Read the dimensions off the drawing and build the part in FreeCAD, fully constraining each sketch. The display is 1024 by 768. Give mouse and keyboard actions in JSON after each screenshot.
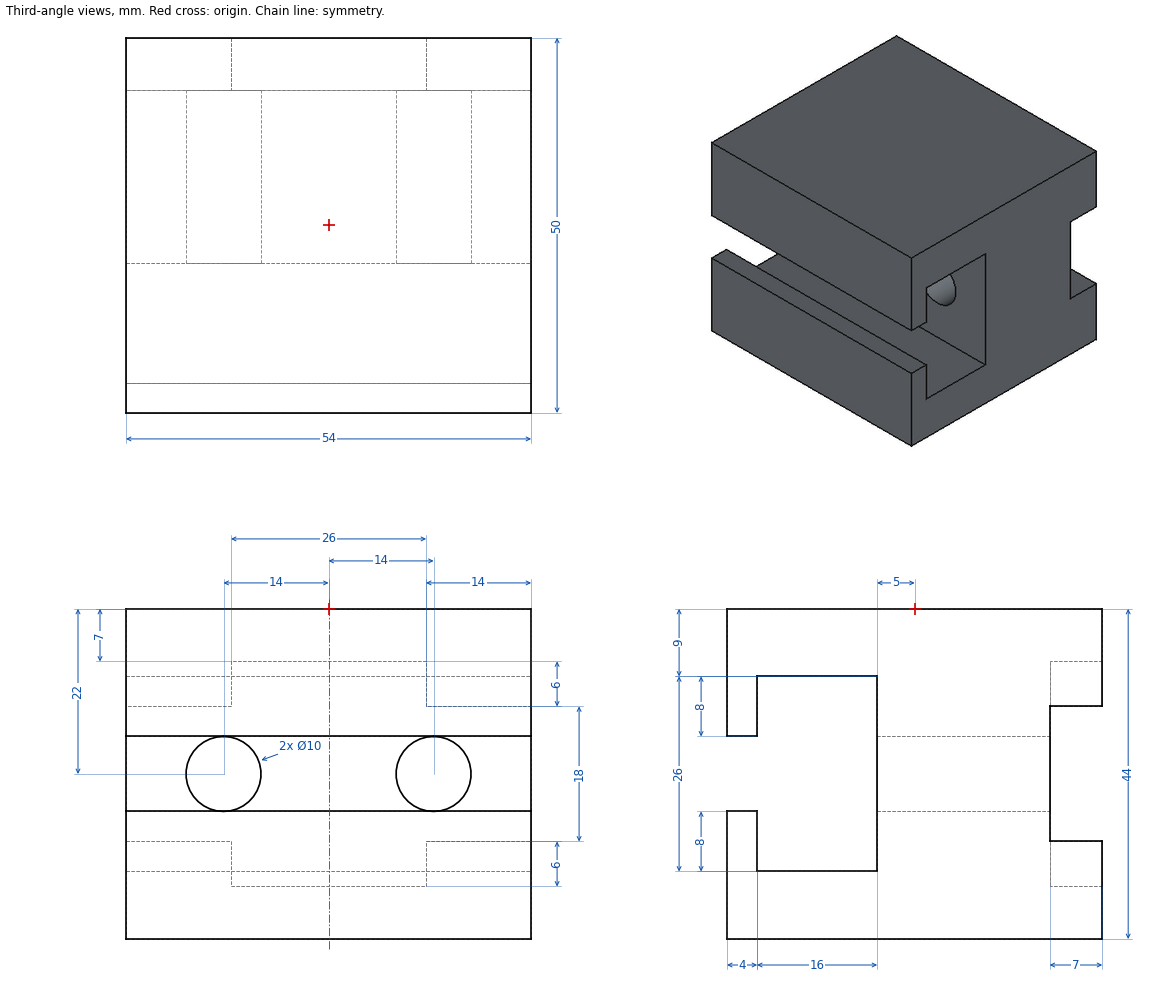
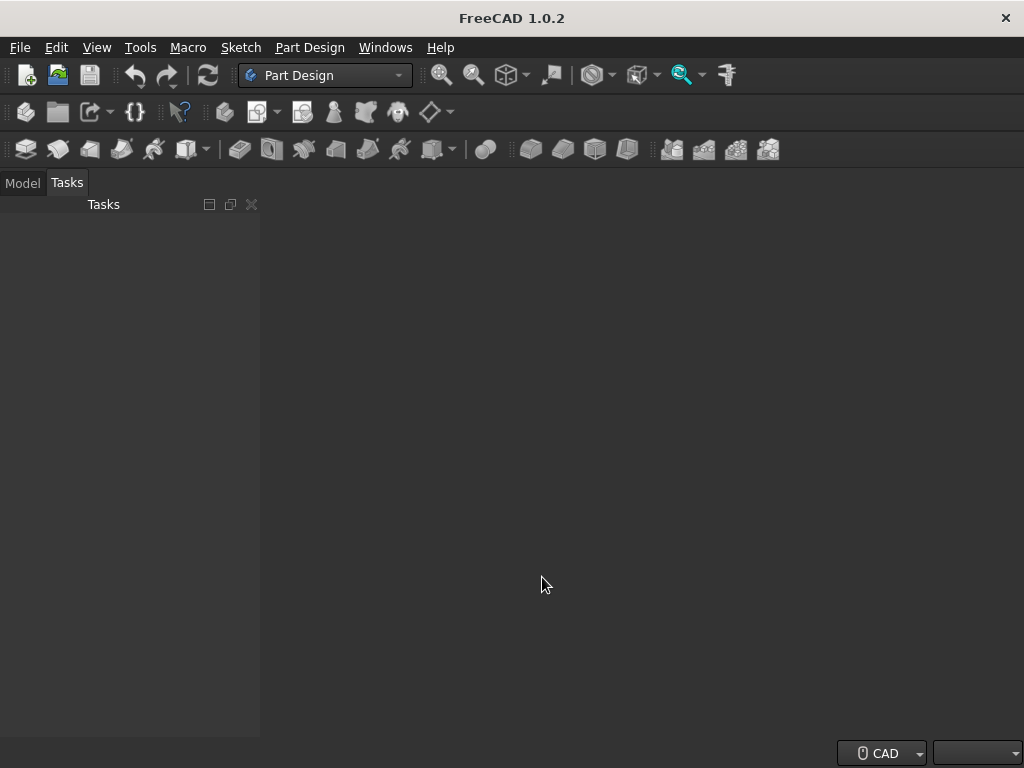
{"action": "key", "text": "ctrl+n"}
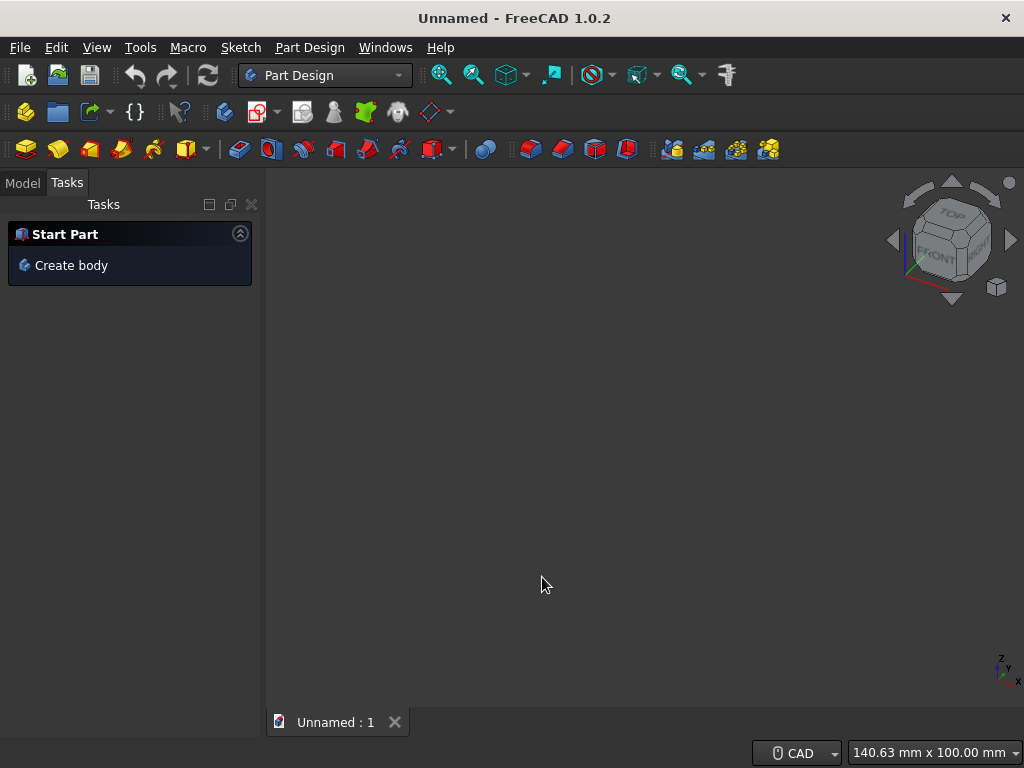
{"action": "left_click", "coordinate": [258, 112]}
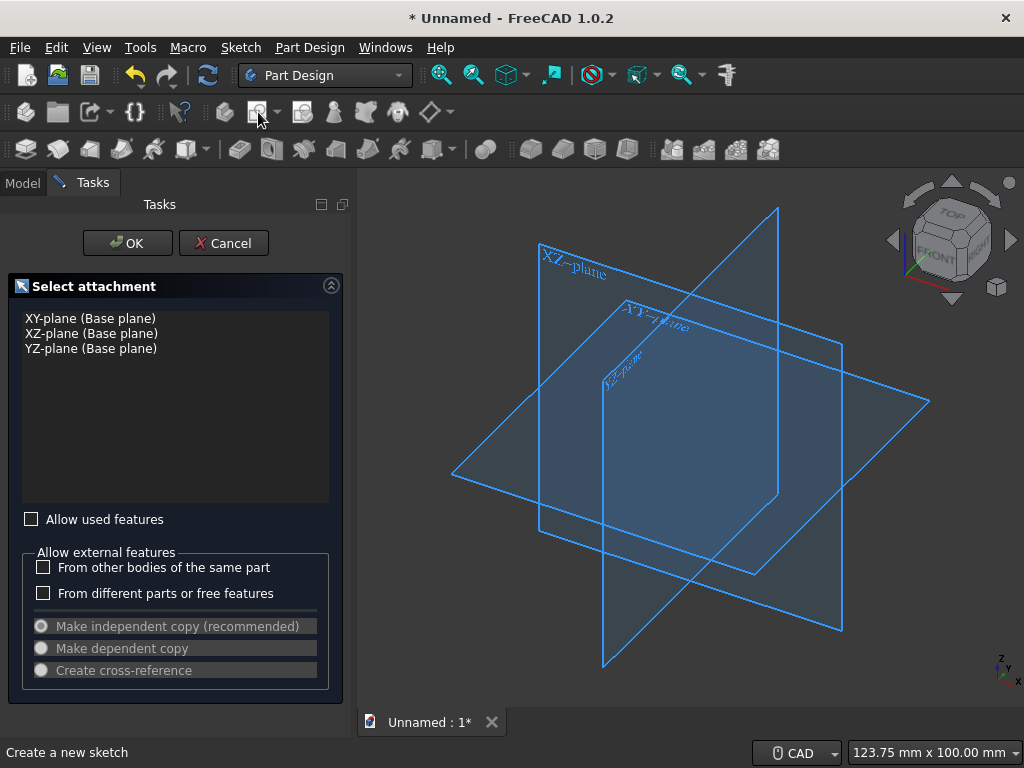
{"action": "left_click", "coordinate": [82, 318]}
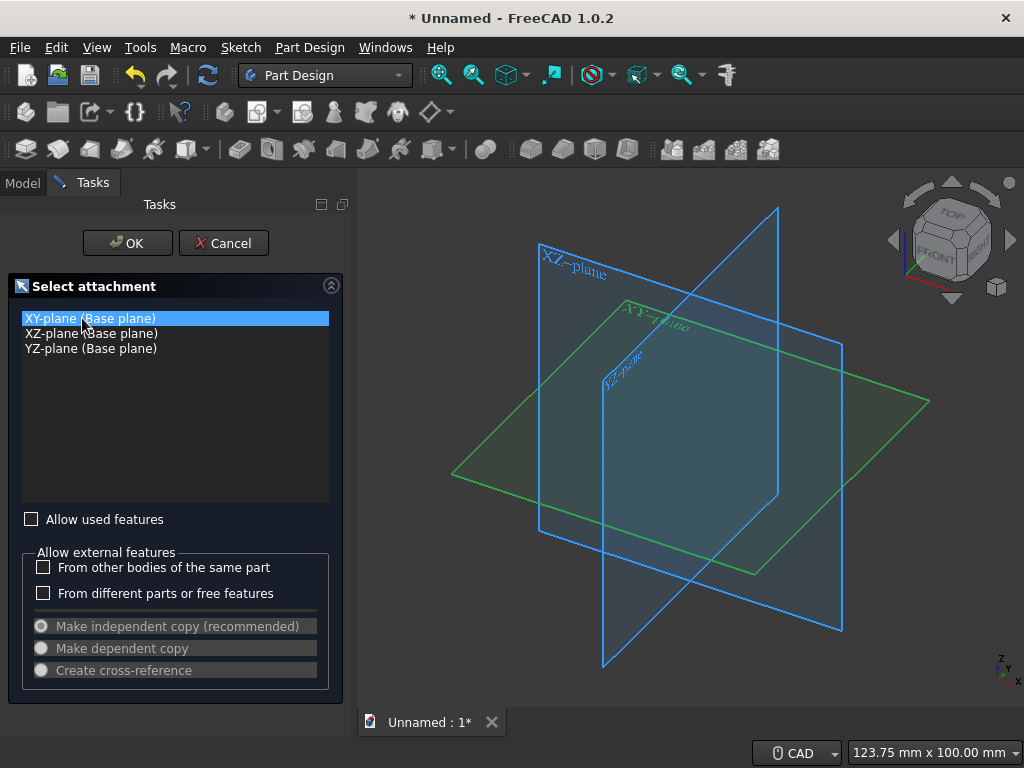
{"action": "left_click", "coordinate": [128, 243]}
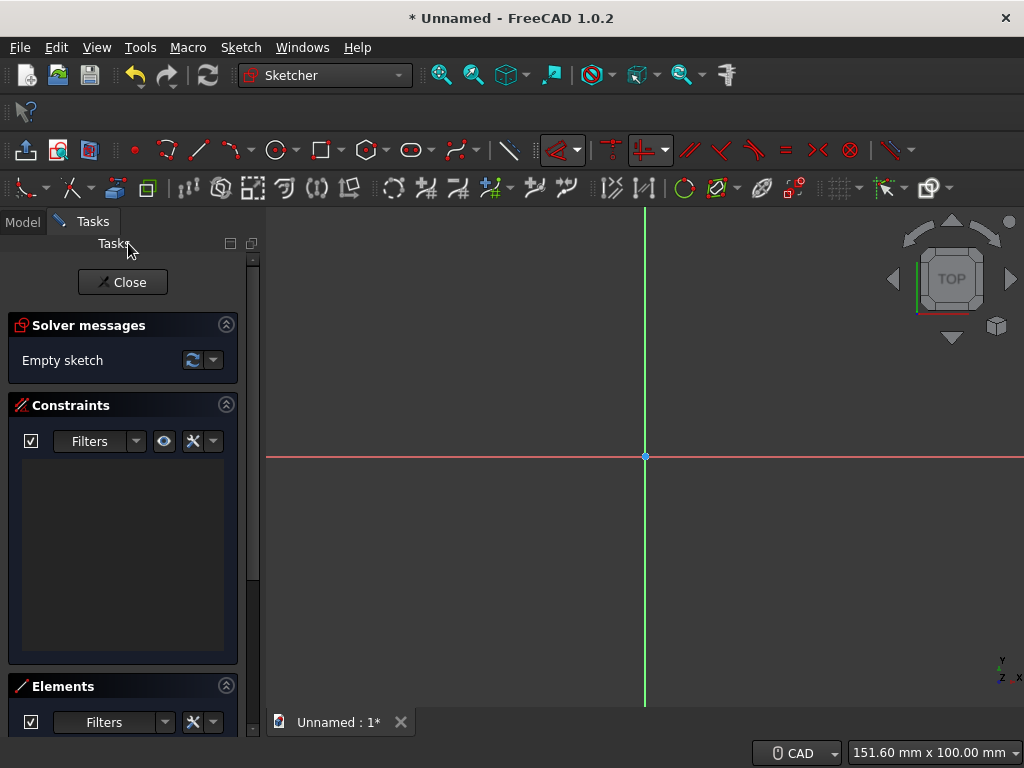
{"action": "key", "text": "g v"}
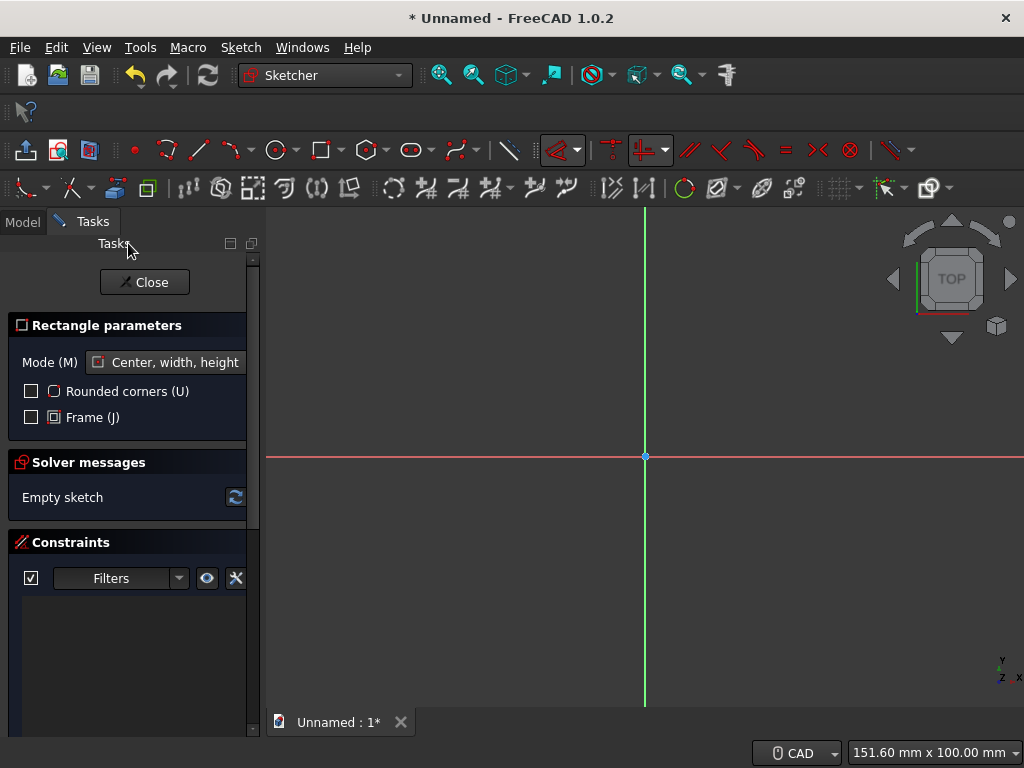
{"action": "left_click", "coordinate": [645, 457]}
{"action": "mouse_move", "coordinate": [780, 332]}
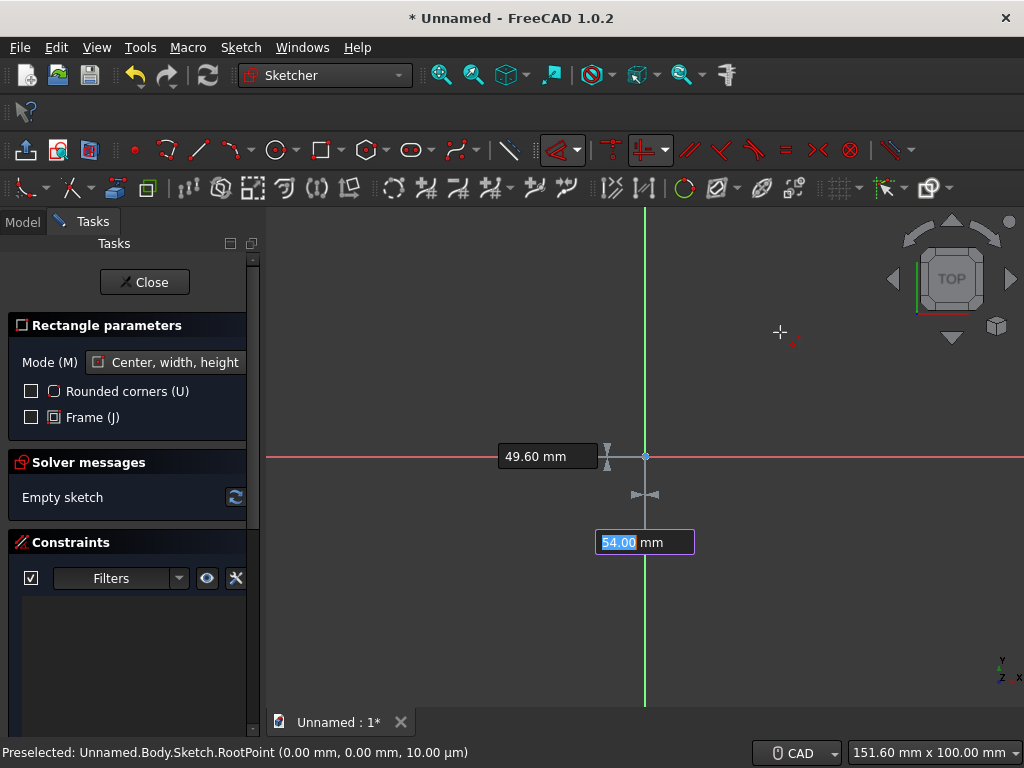
{"action": "type", "text": "54"}
{"action": "key", "text": "Tab"}
{"action": "type", "text": "50"}
{"action": "key", "text": "Return"}
{"action": "key", "text": "Escape"}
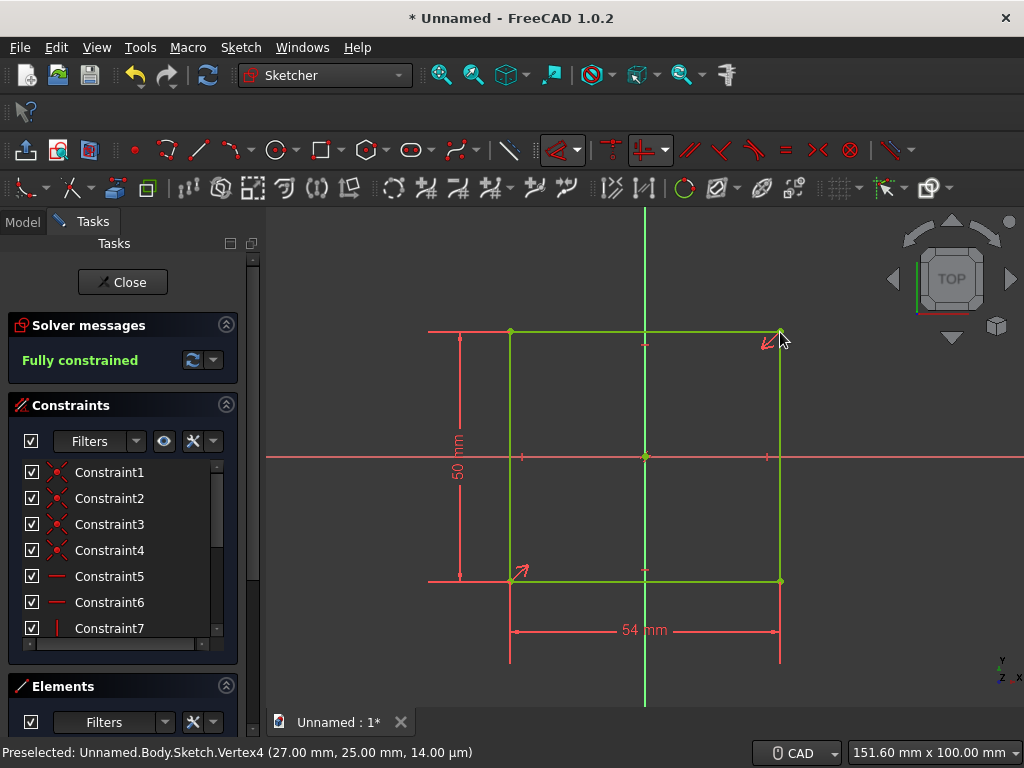
{"action": "left_click", "coordinate": [123, 282]}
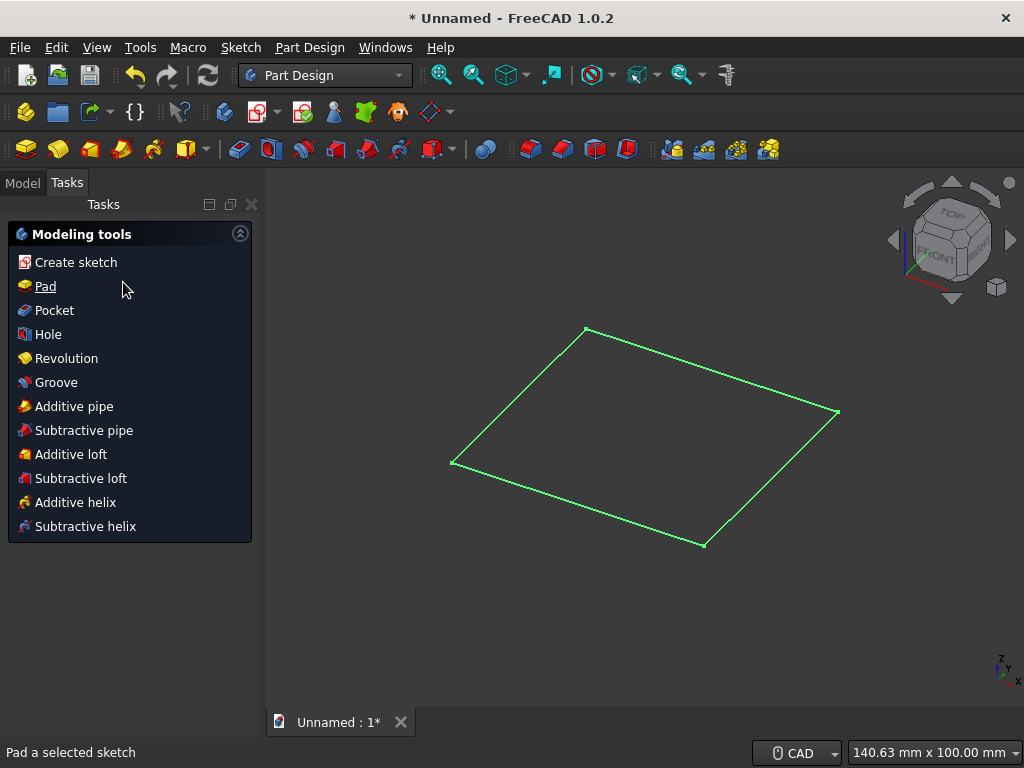
{"action": "left_click", "coordinate": [26, 150]}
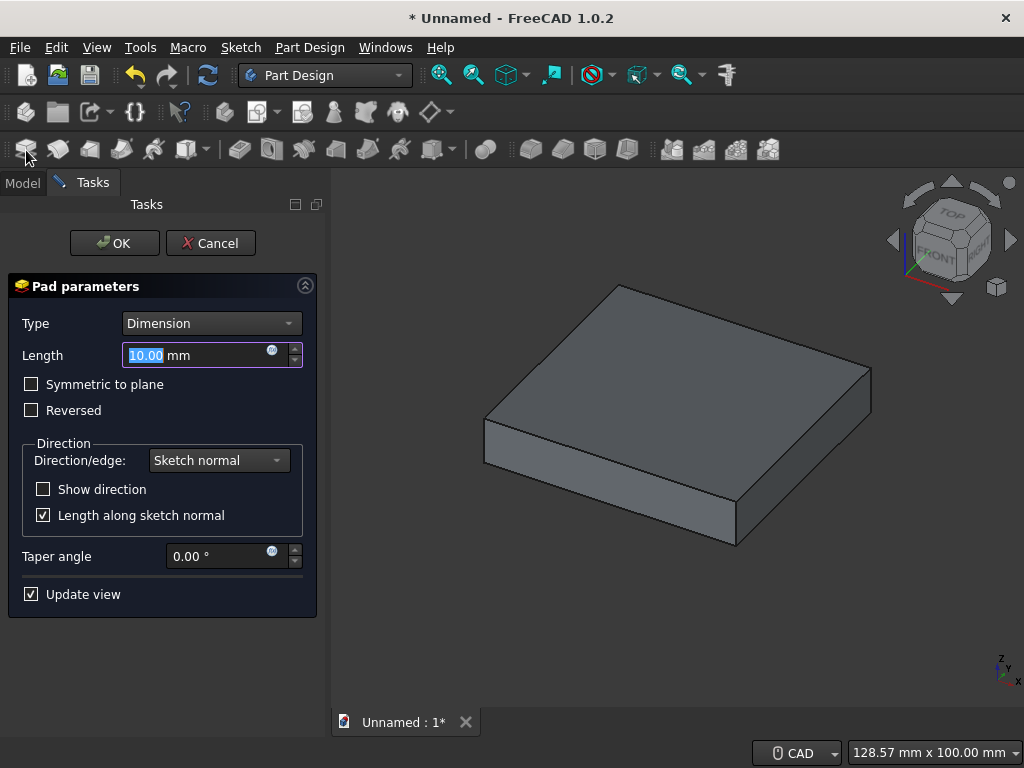
{"action": "type", "text": "44"}
{"action": "key", "text": "Tab"}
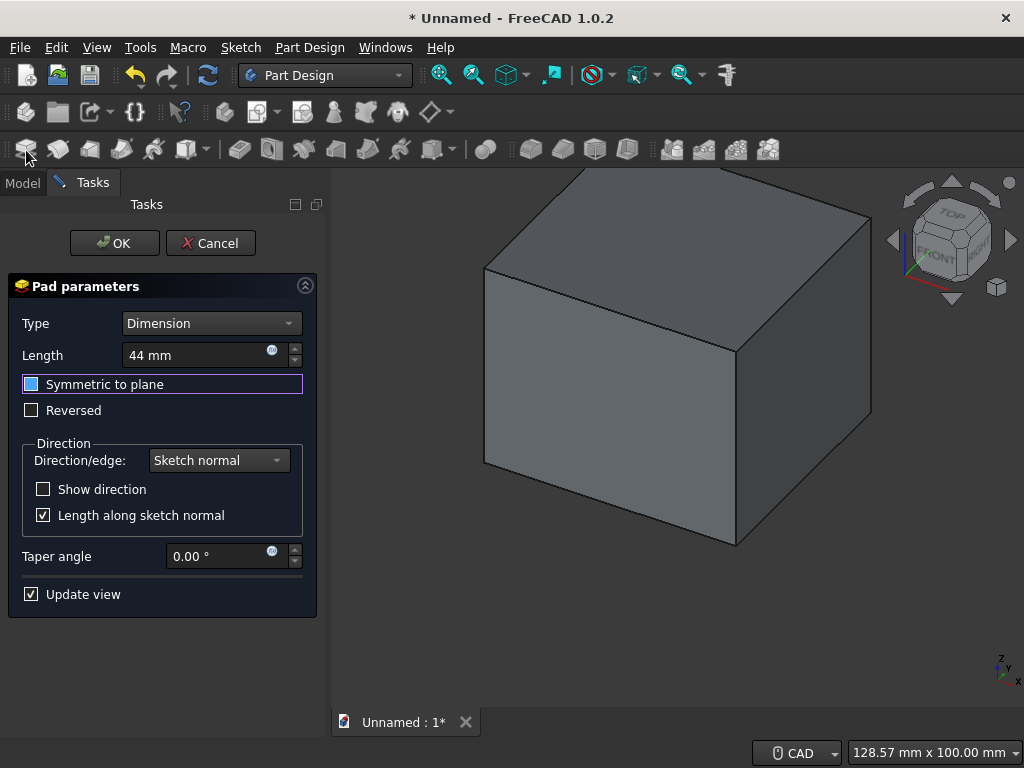
{"action": "left_click", "coordinate": [30, 410]}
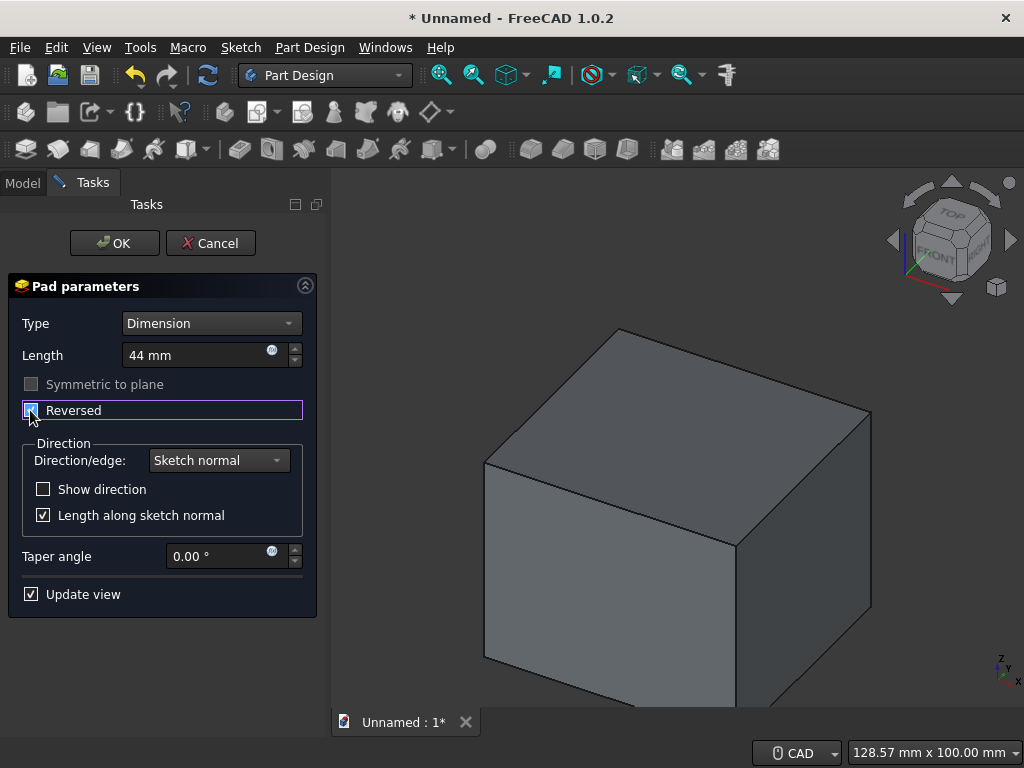
{"action": "left_click", "coordinate": [115, 243]}